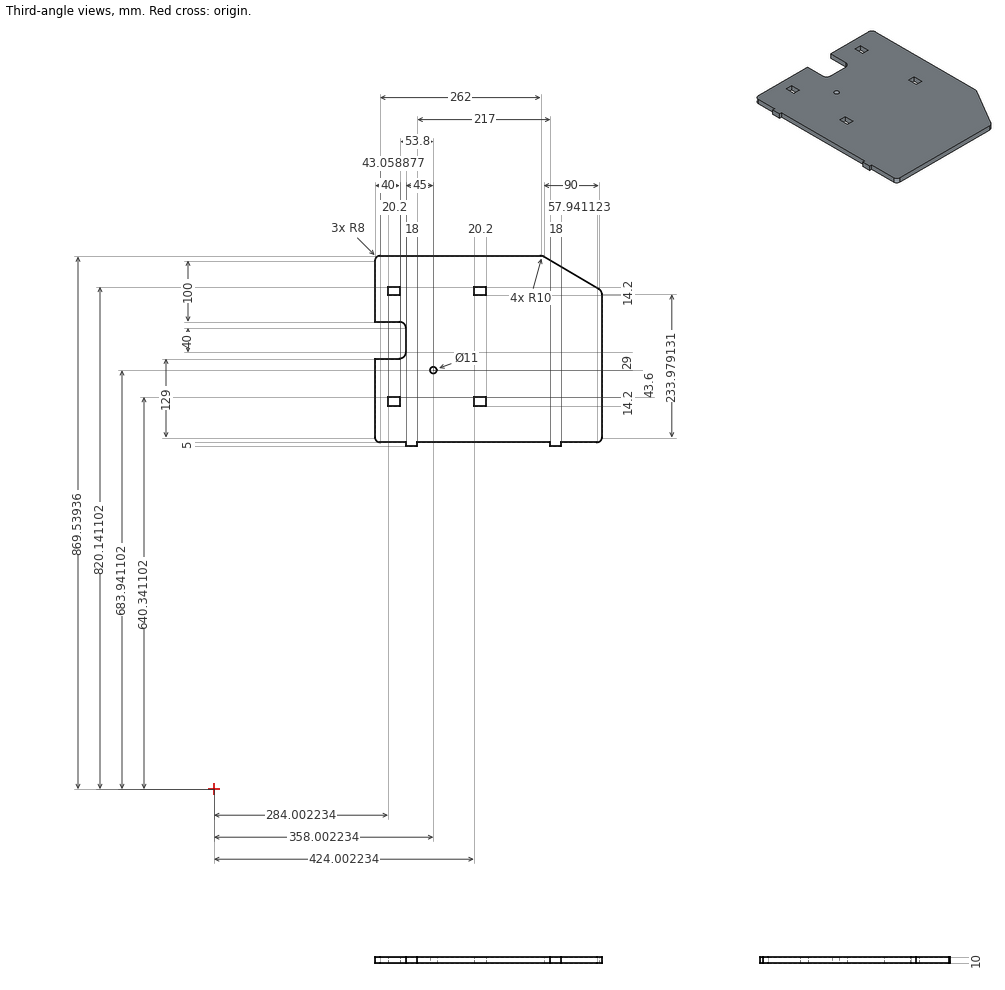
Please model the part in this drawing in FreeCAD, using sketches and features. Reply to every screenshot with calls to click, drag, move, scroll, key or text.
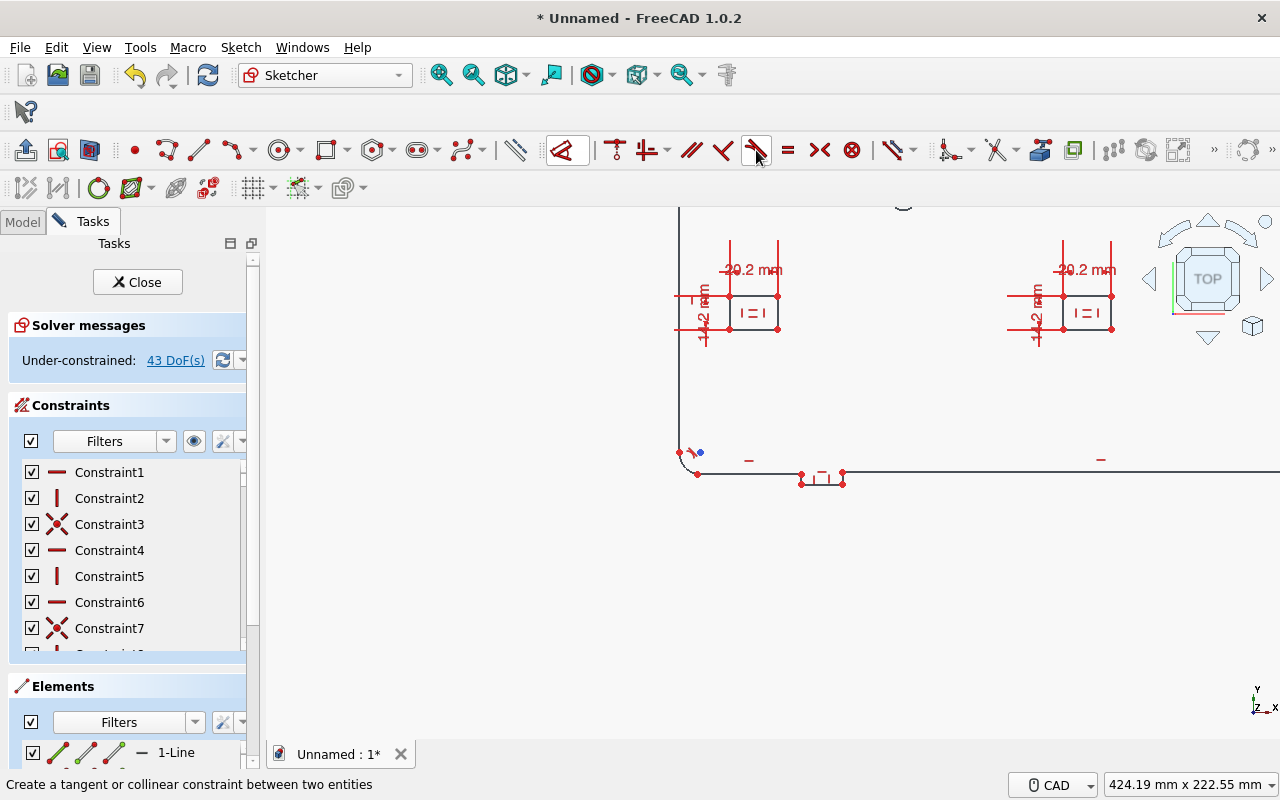
click(729, 474)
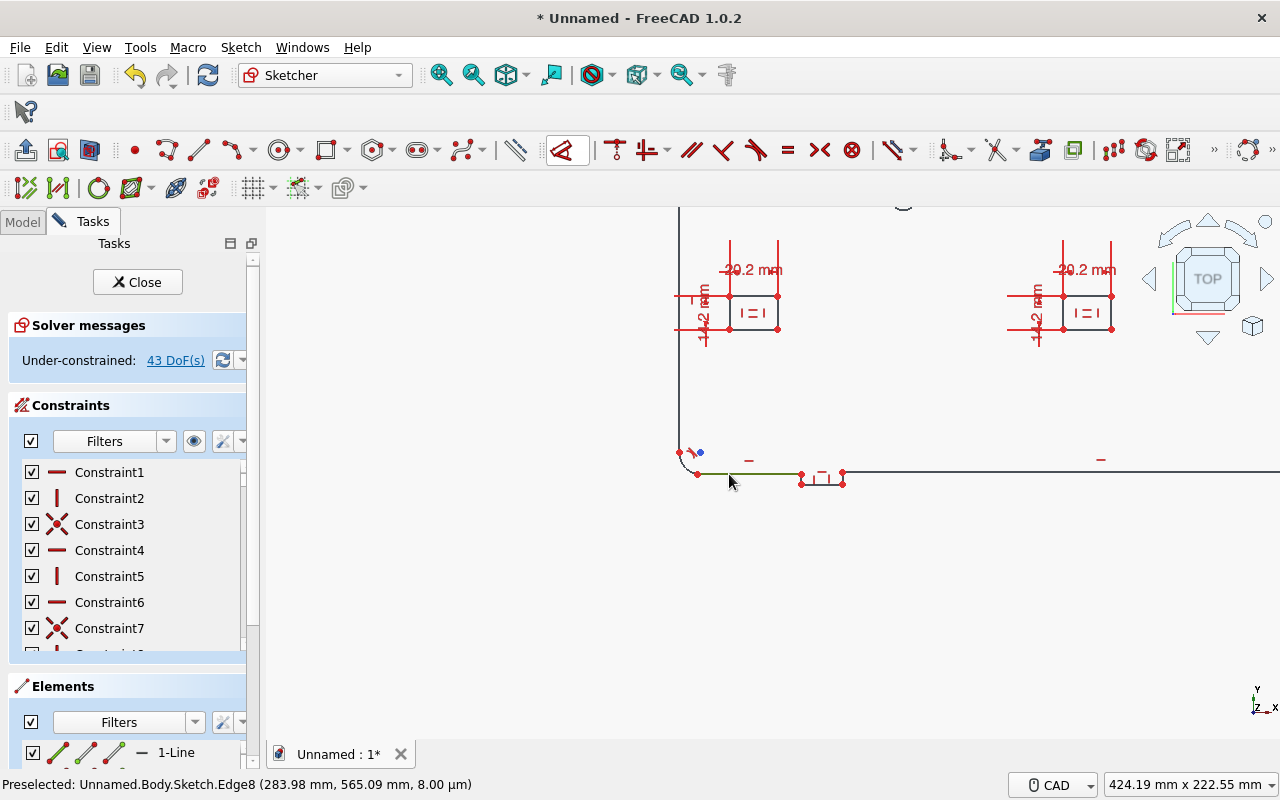
scroll(681, 462, up, 3)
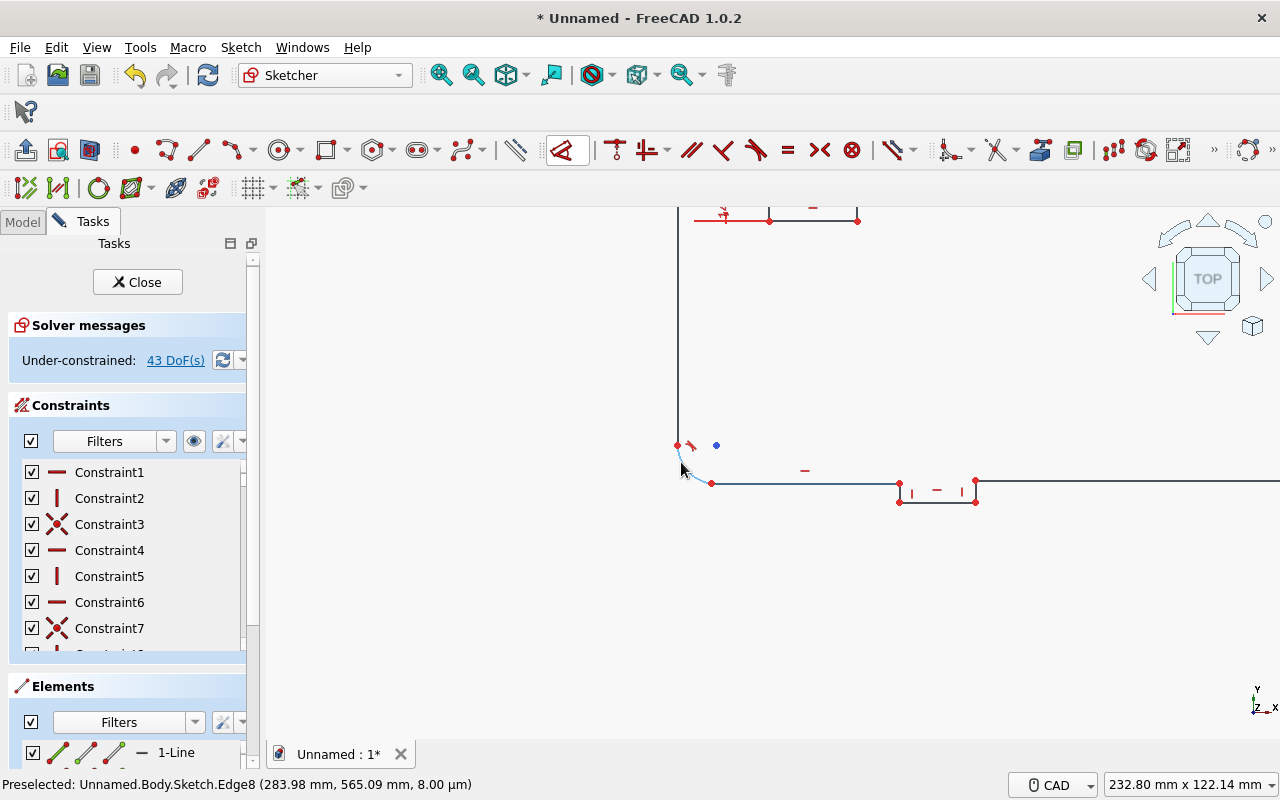
click(681, 461)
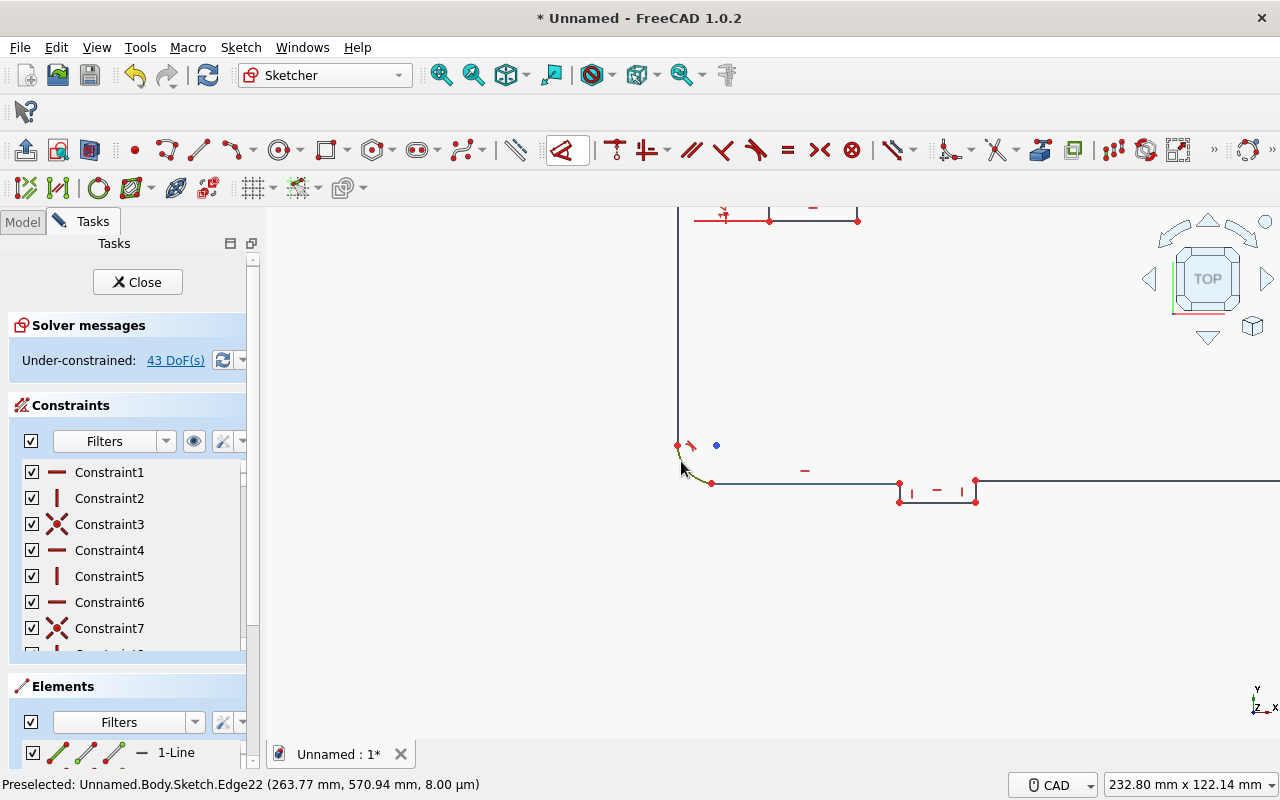
click(756, 150)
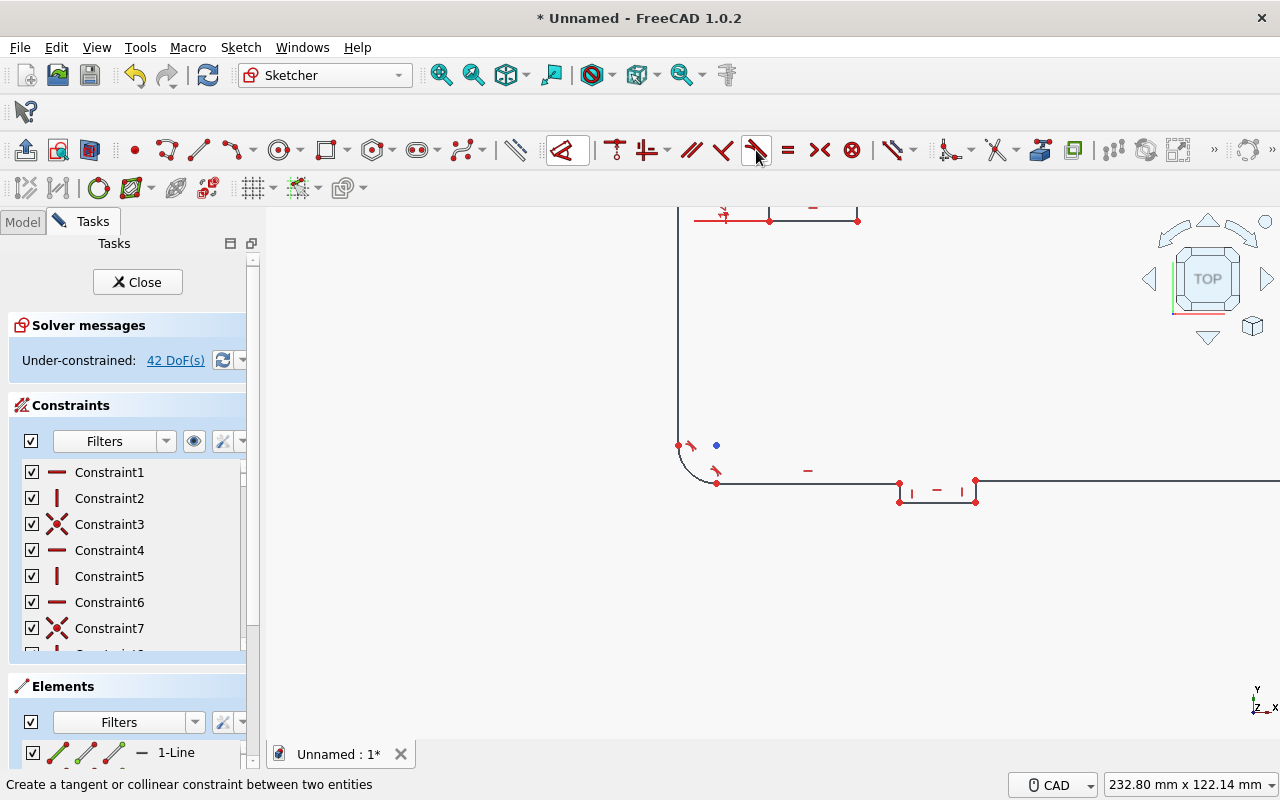
scroll(684, 416, down, 12)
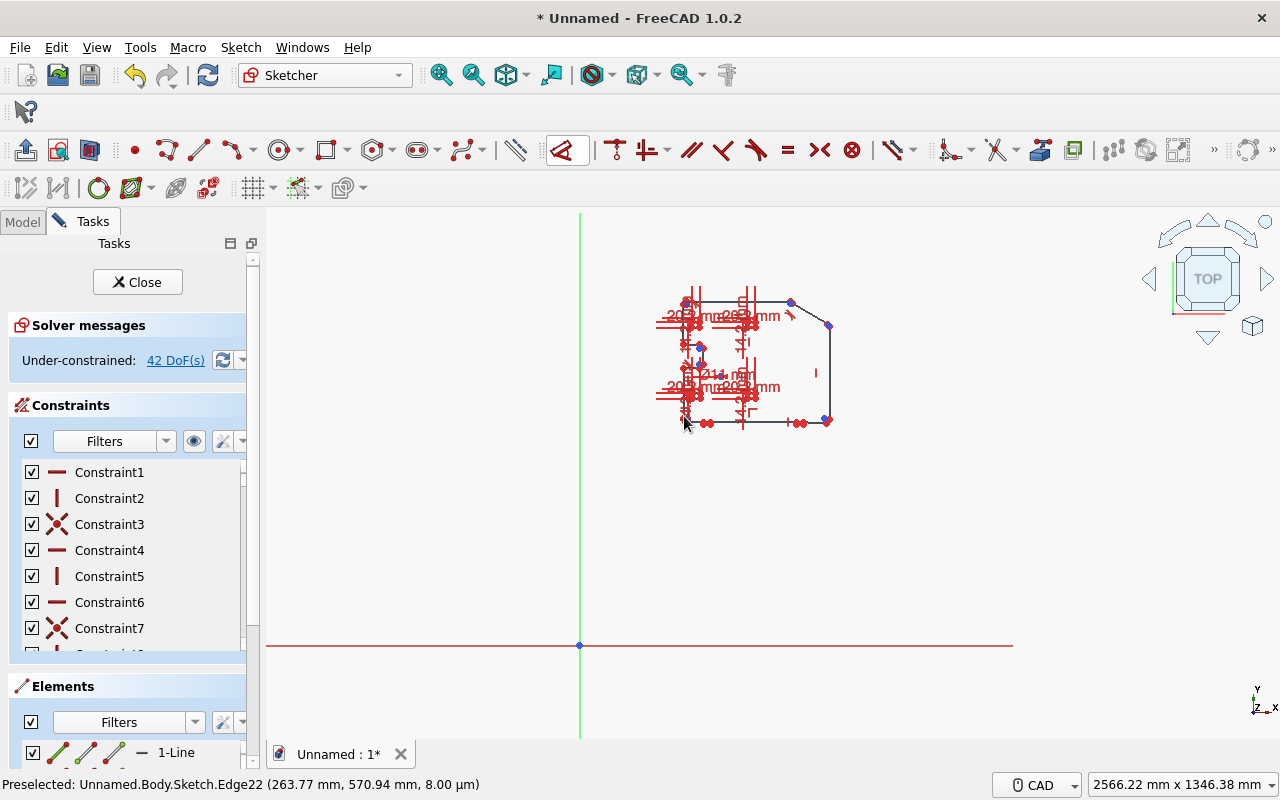
scroll(810, 423, up, 4)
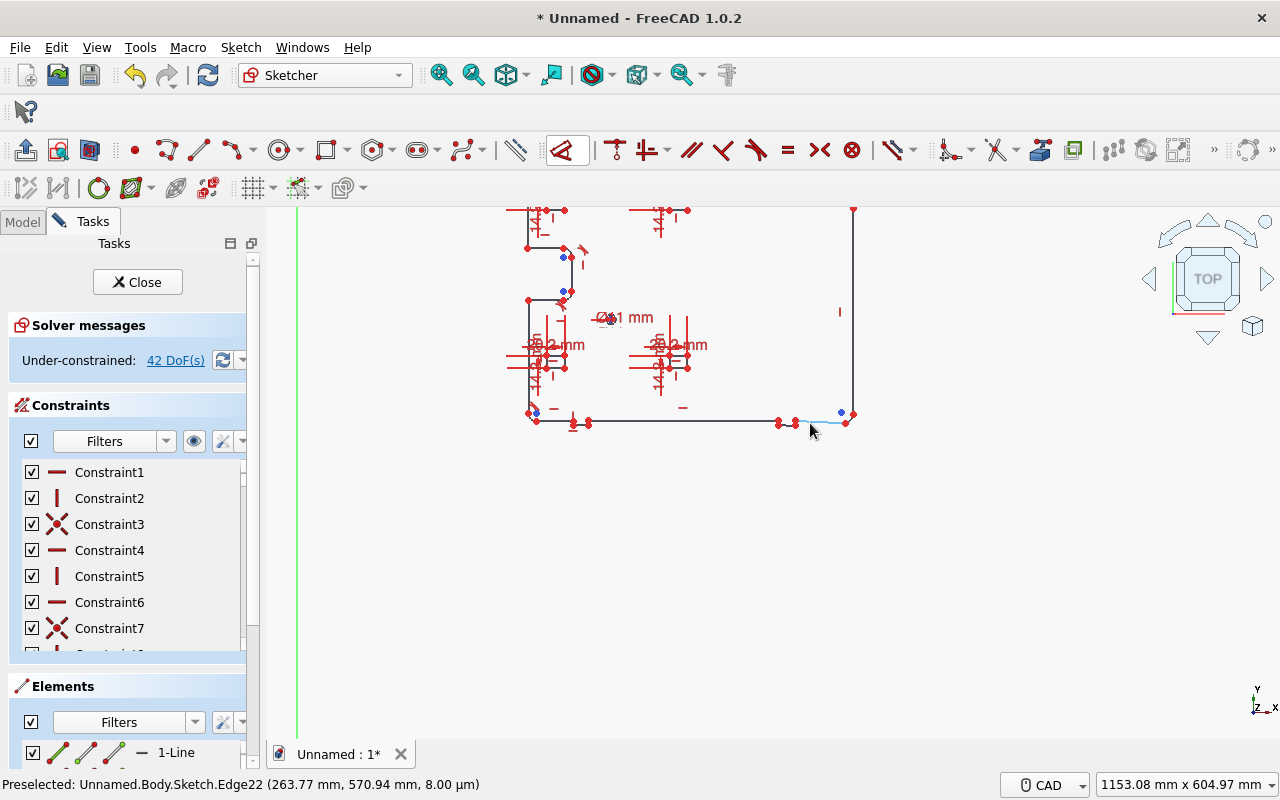
click(810, 422)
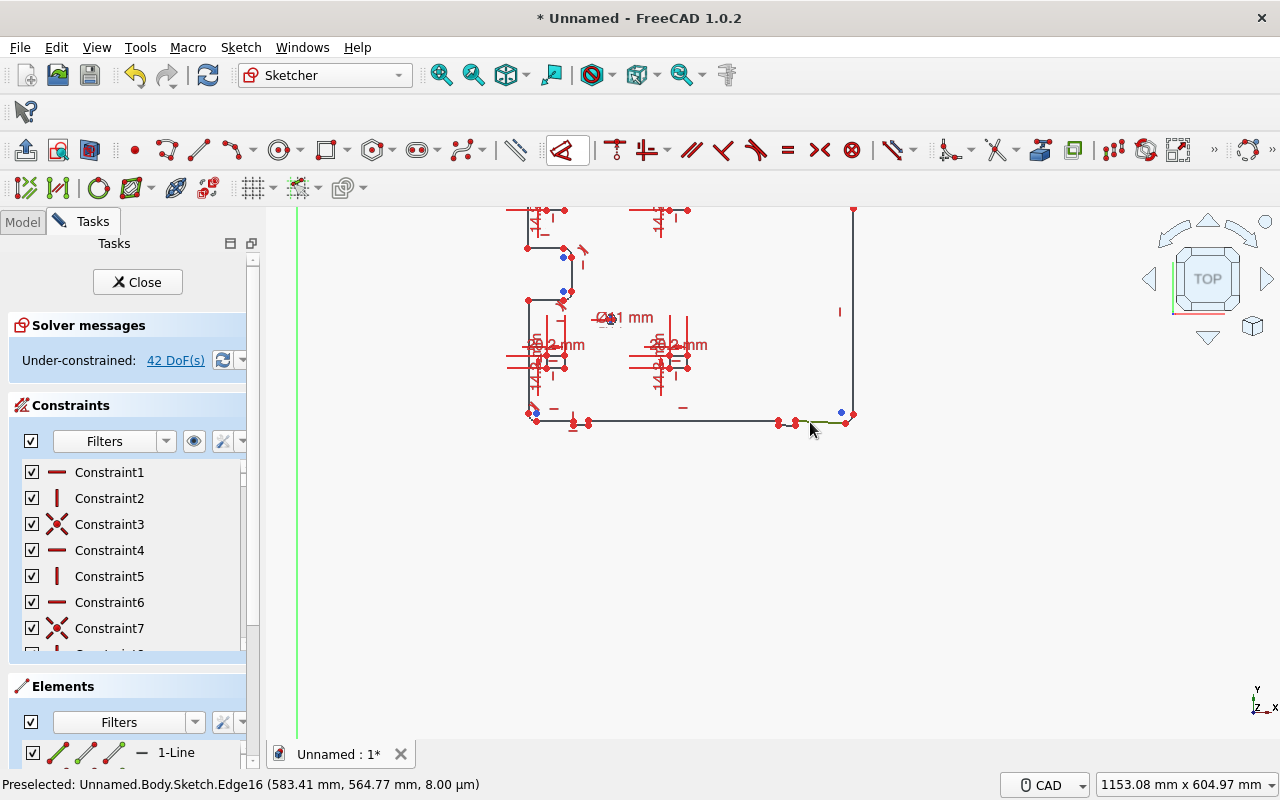
scroll(851, 420, up, 4)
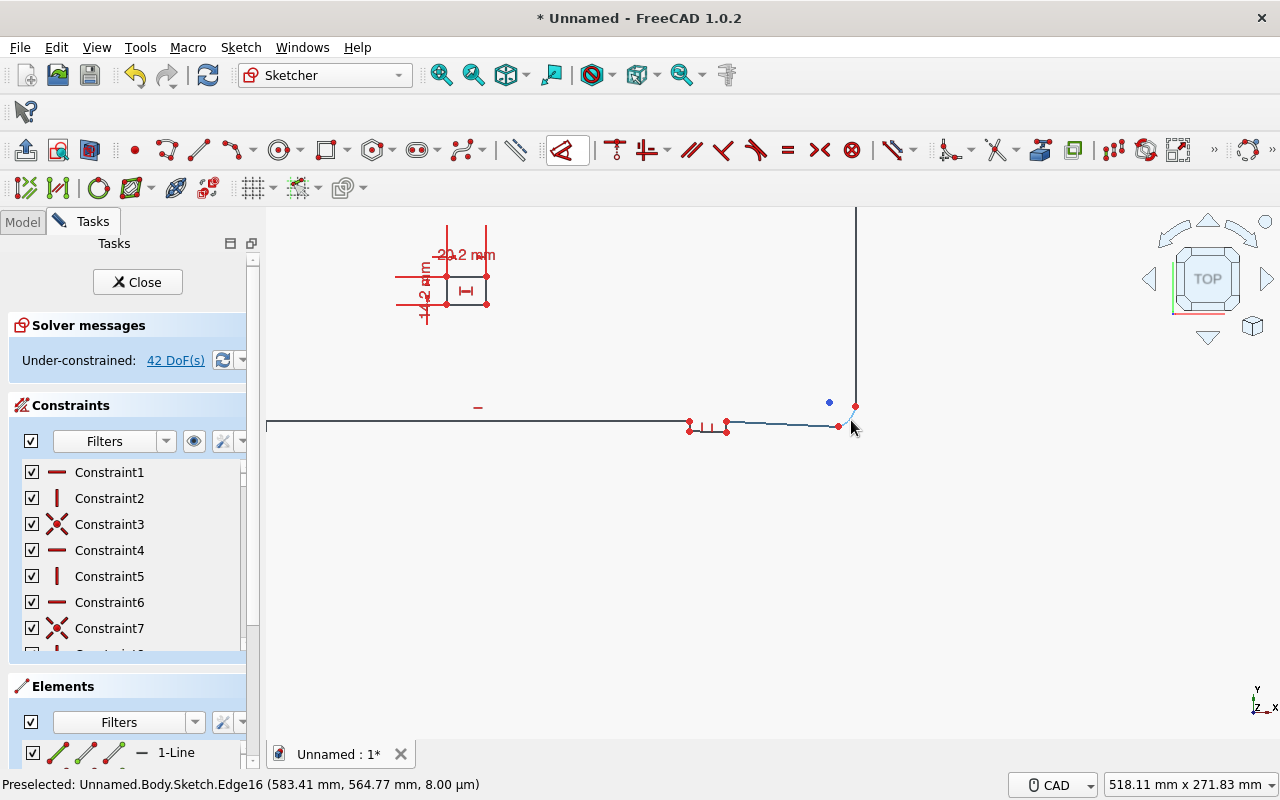
click(850, 419)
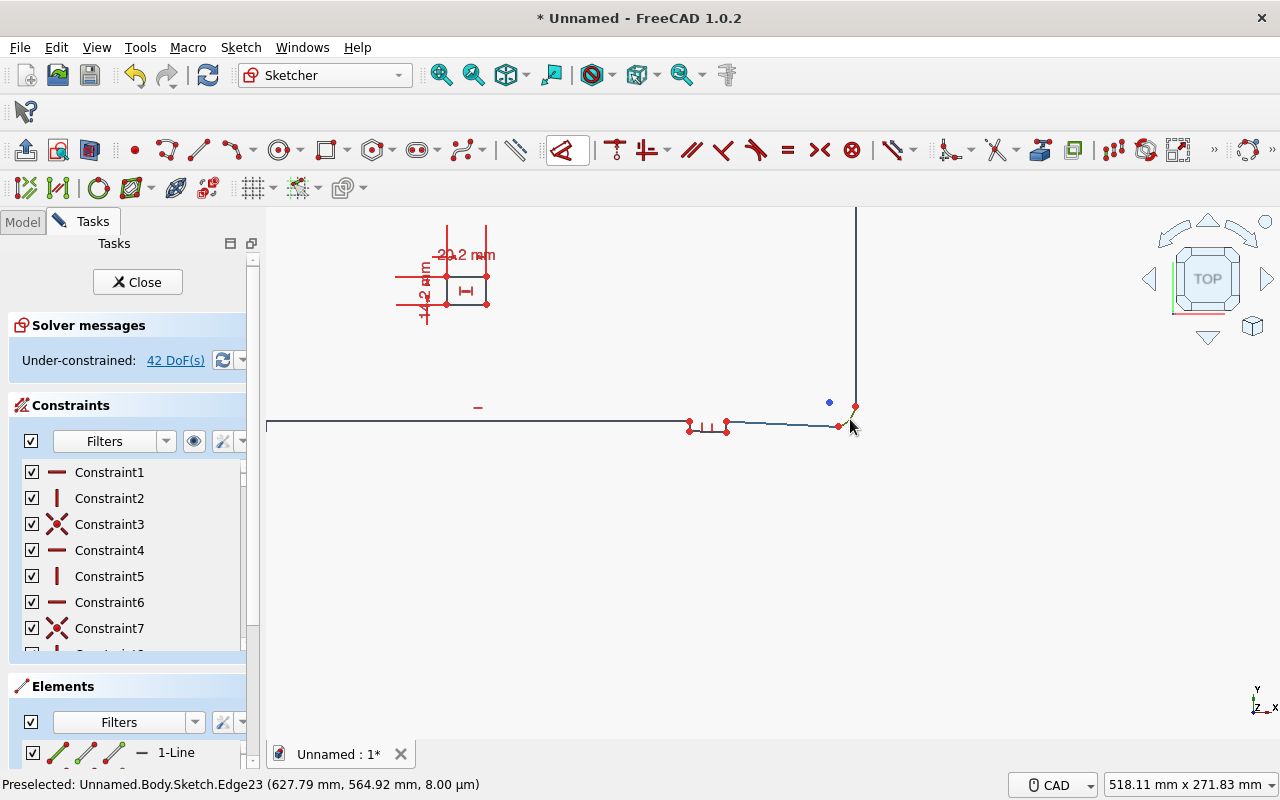
key(t)